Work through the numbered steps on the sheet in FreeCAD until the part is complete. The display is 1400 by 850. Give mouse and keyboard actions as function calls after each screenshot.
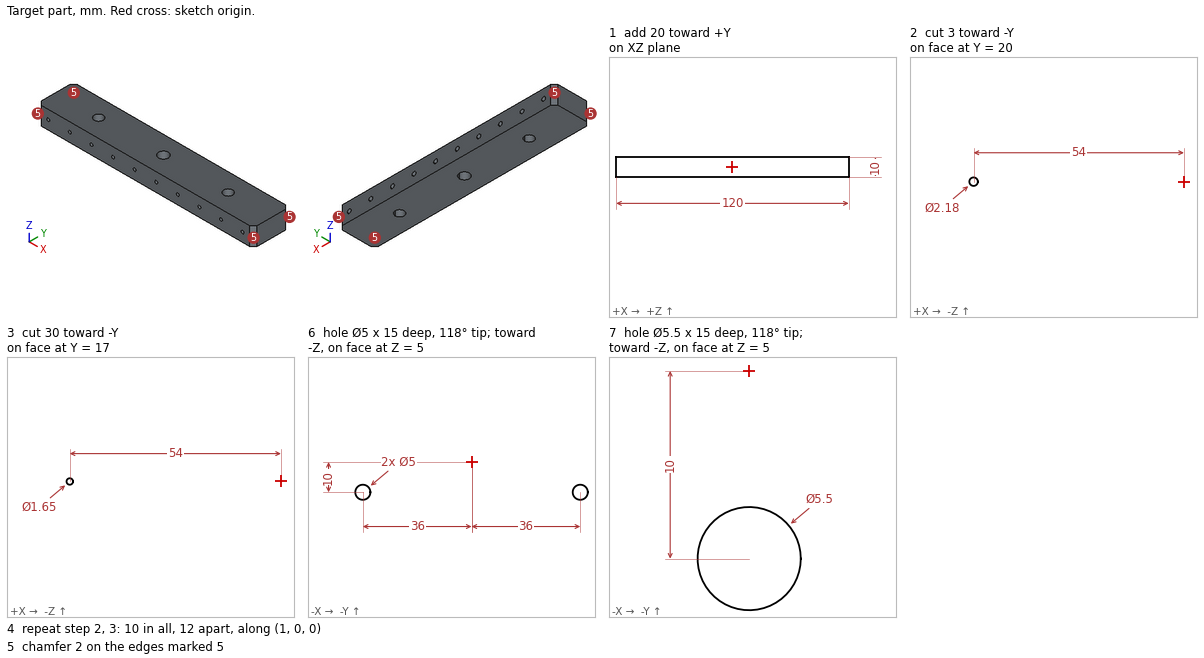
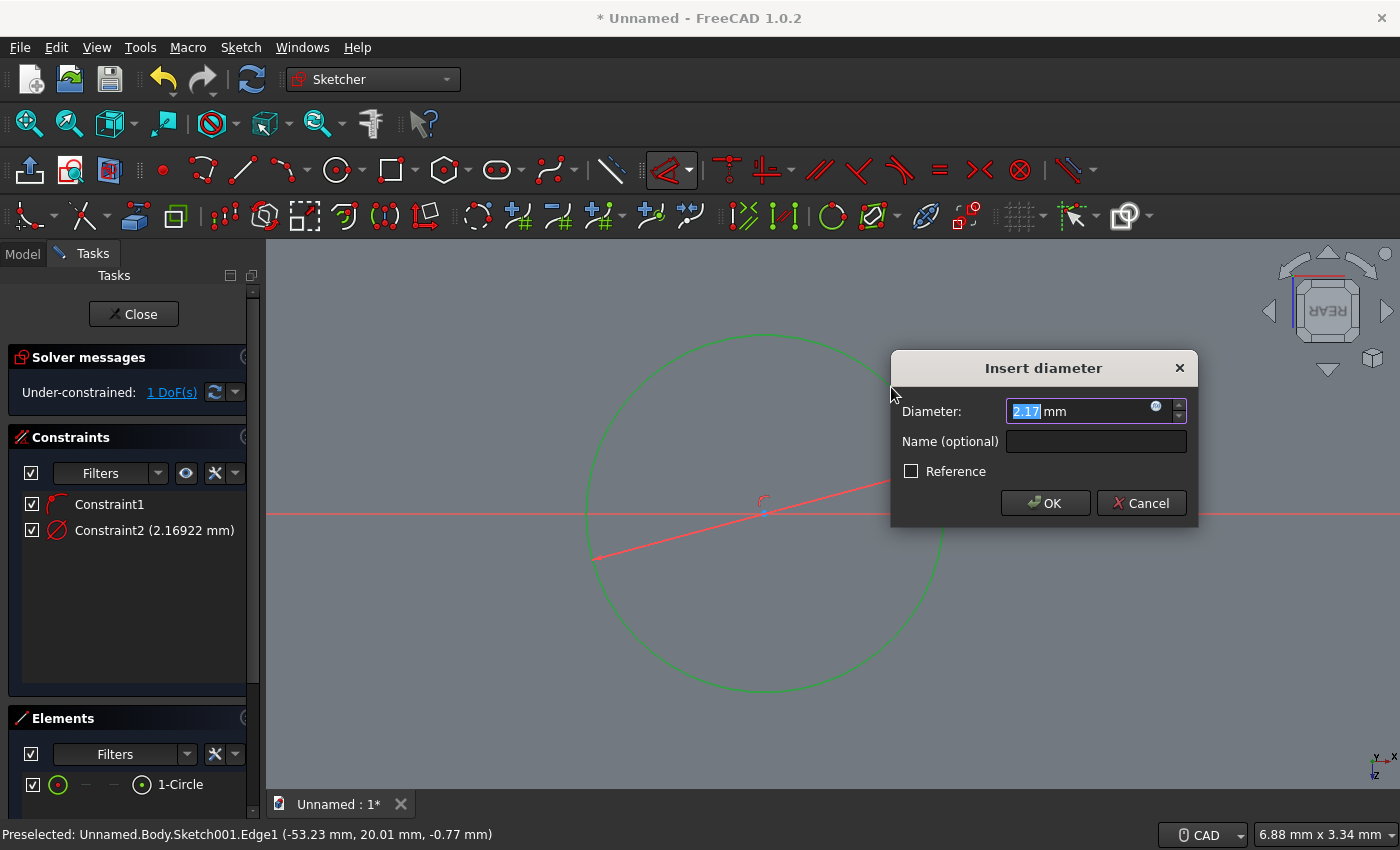
text(2.18)
key(Return)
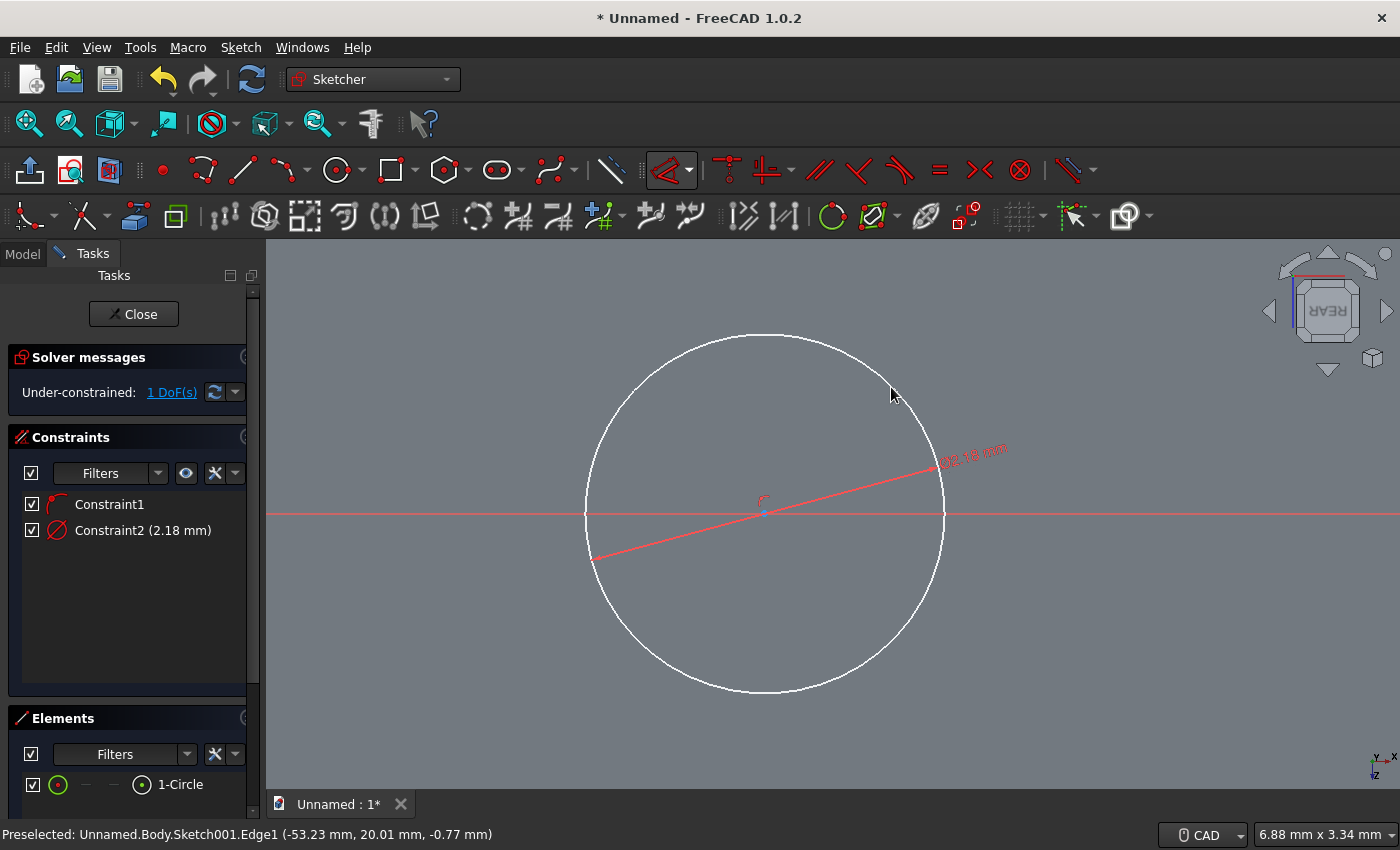
click(765, 514)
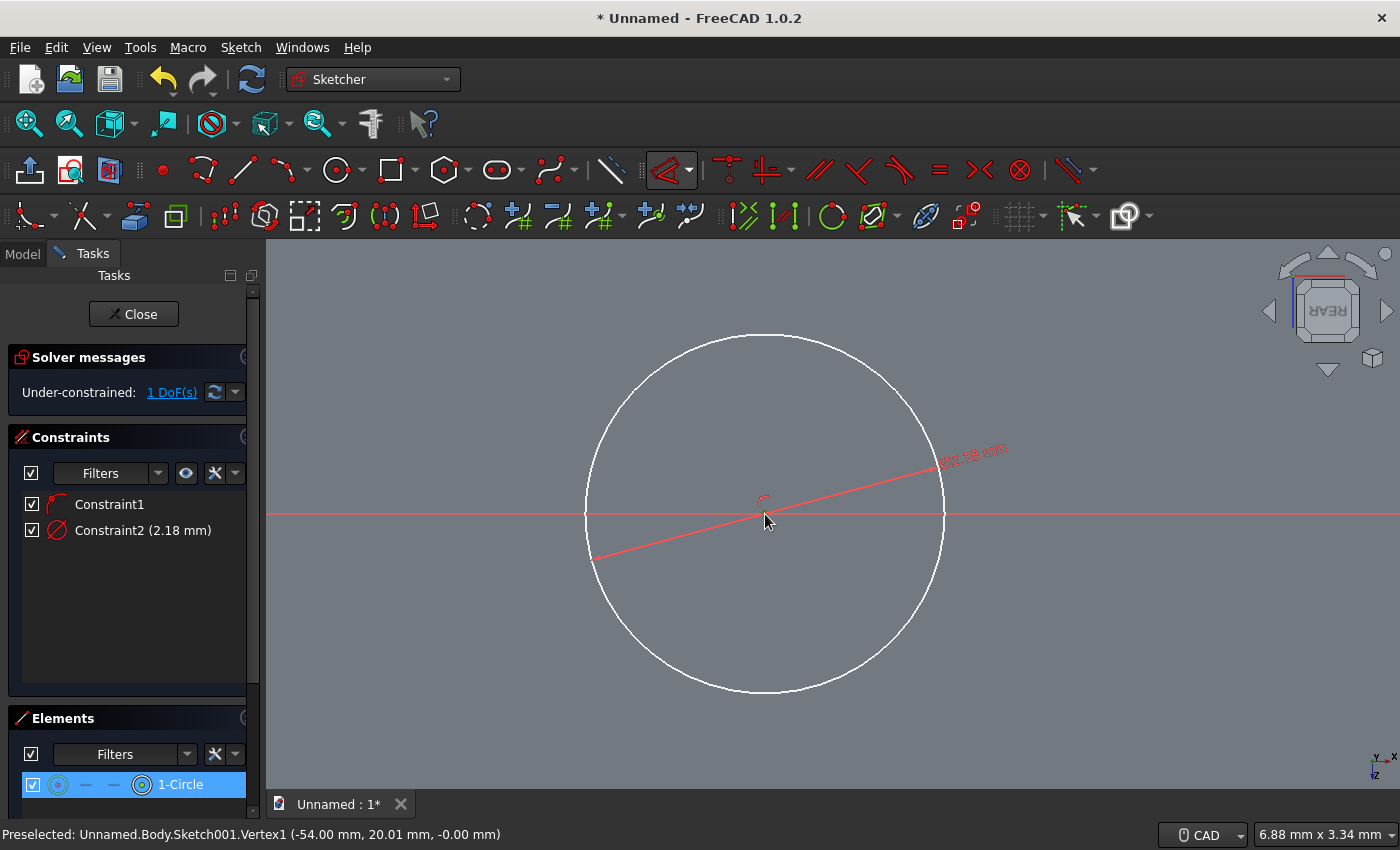
click(692, 170)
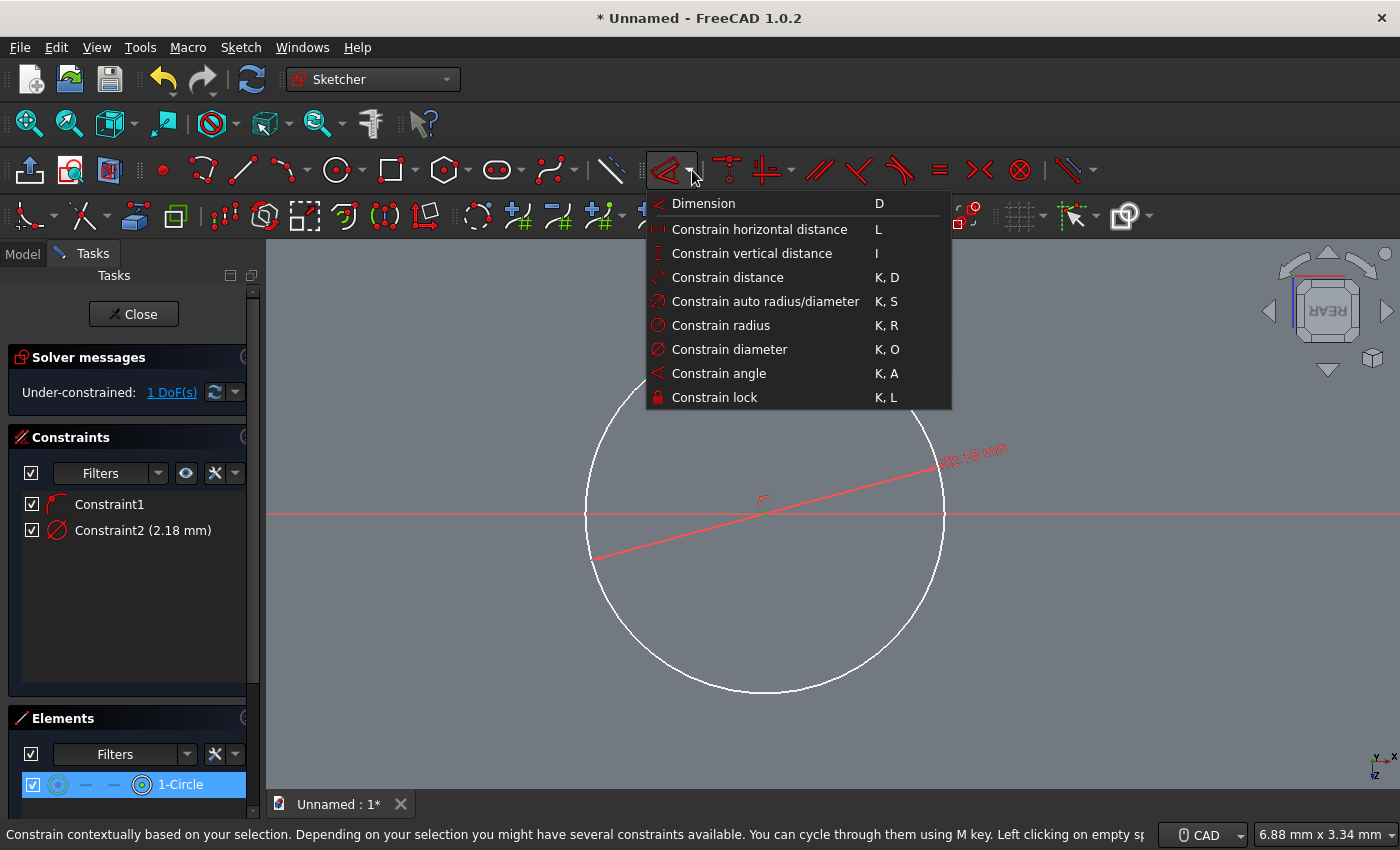
click(799, 229)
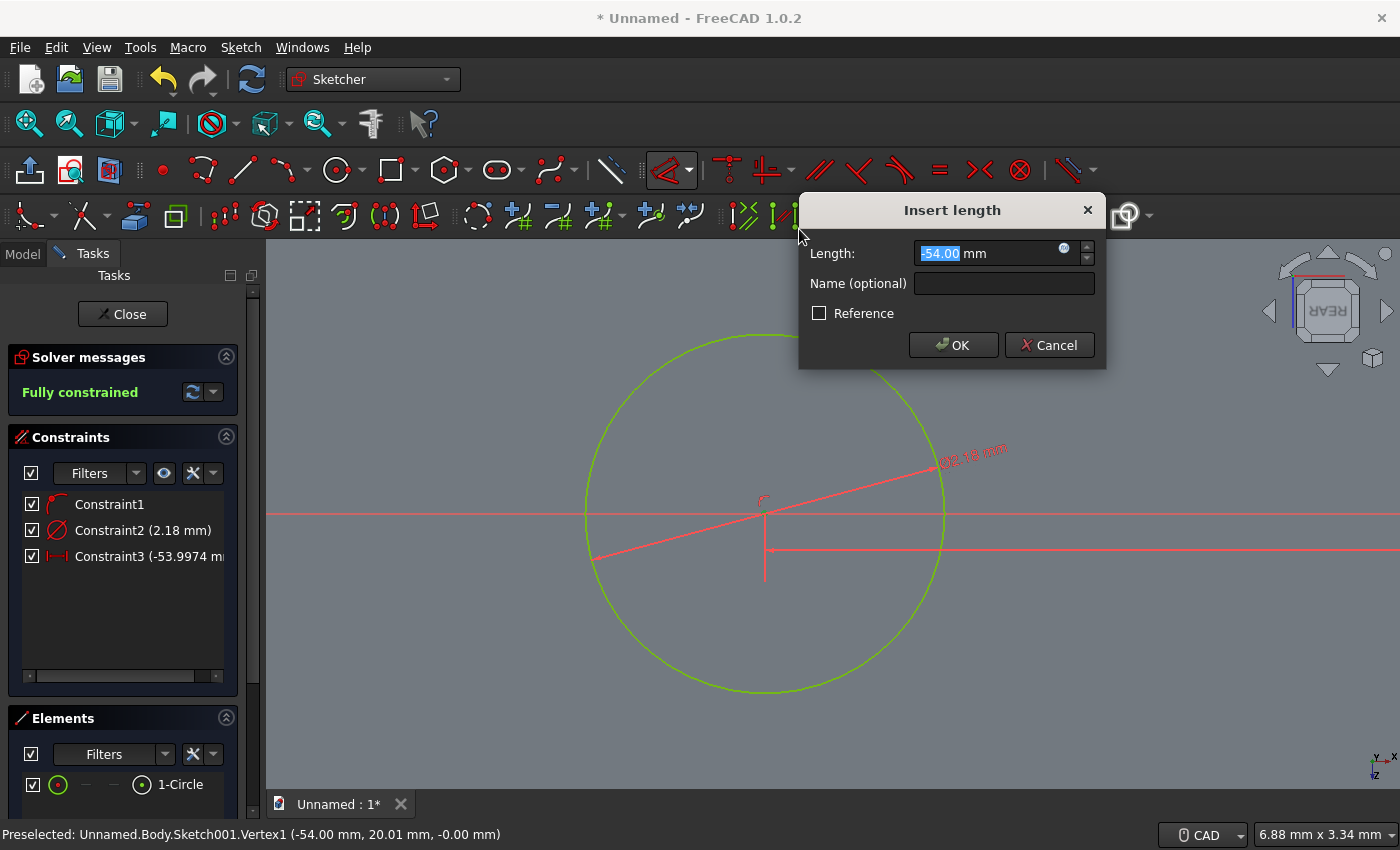
text(-54)
key(Return)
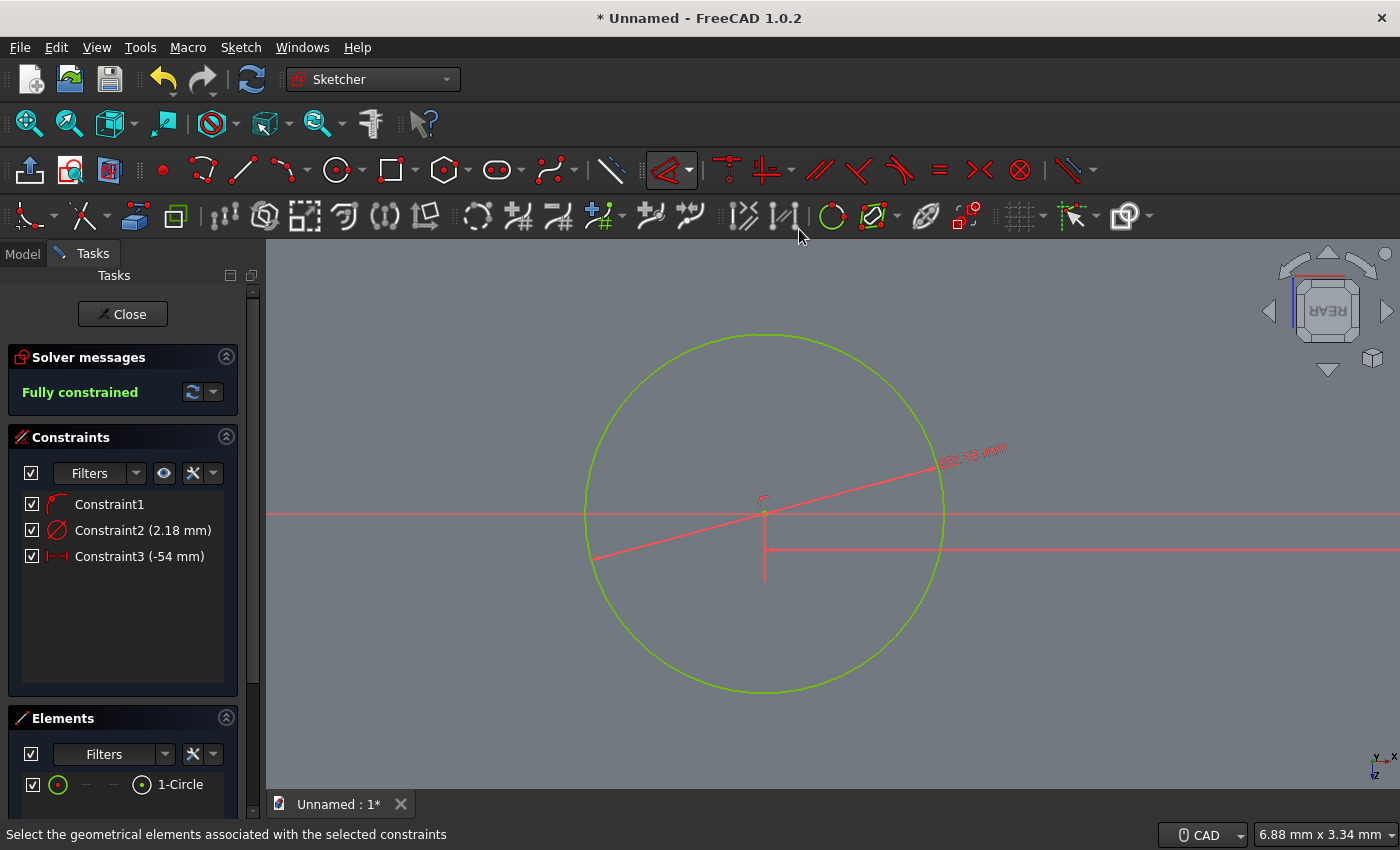
click(123, 314)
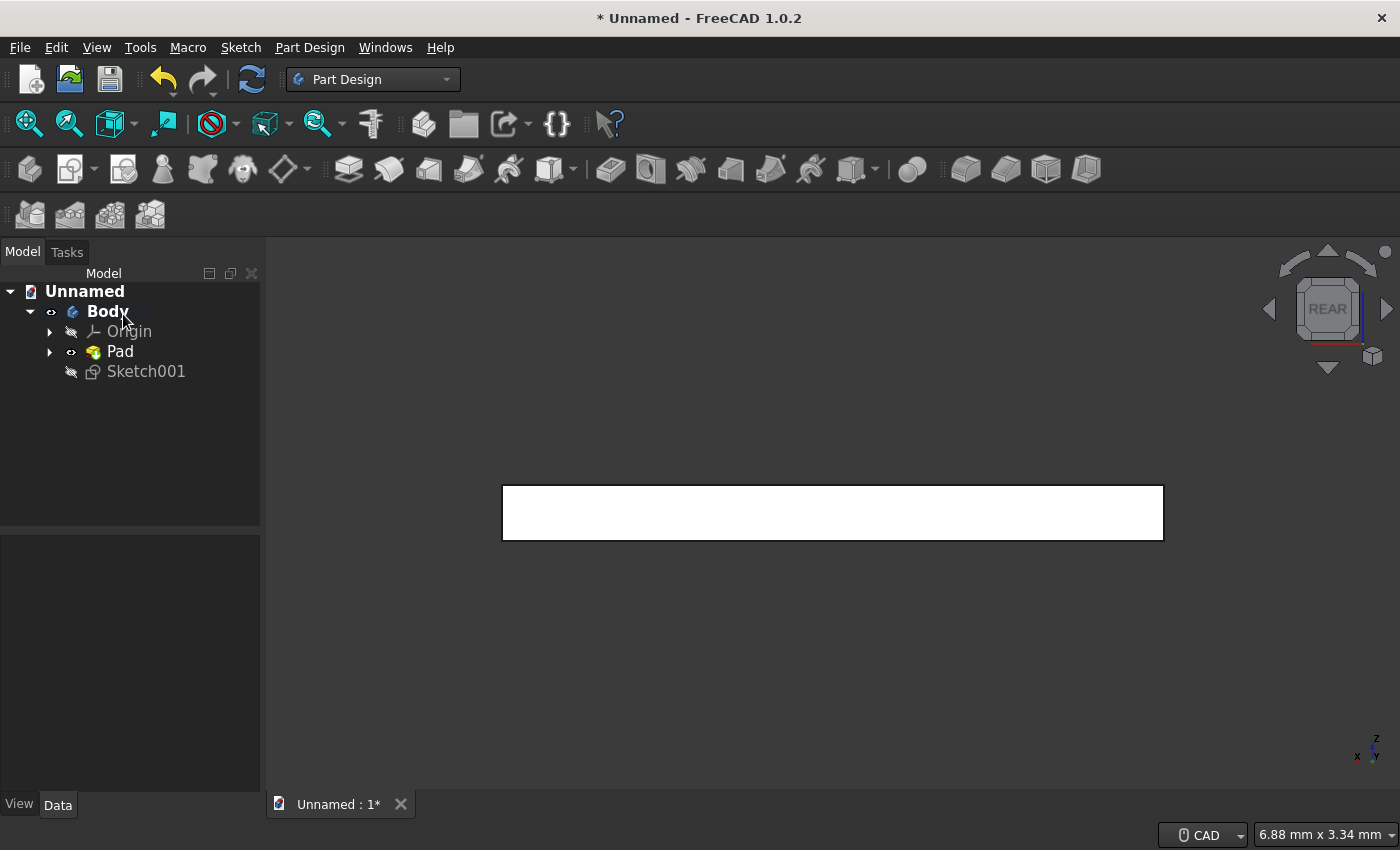
click(612, 170)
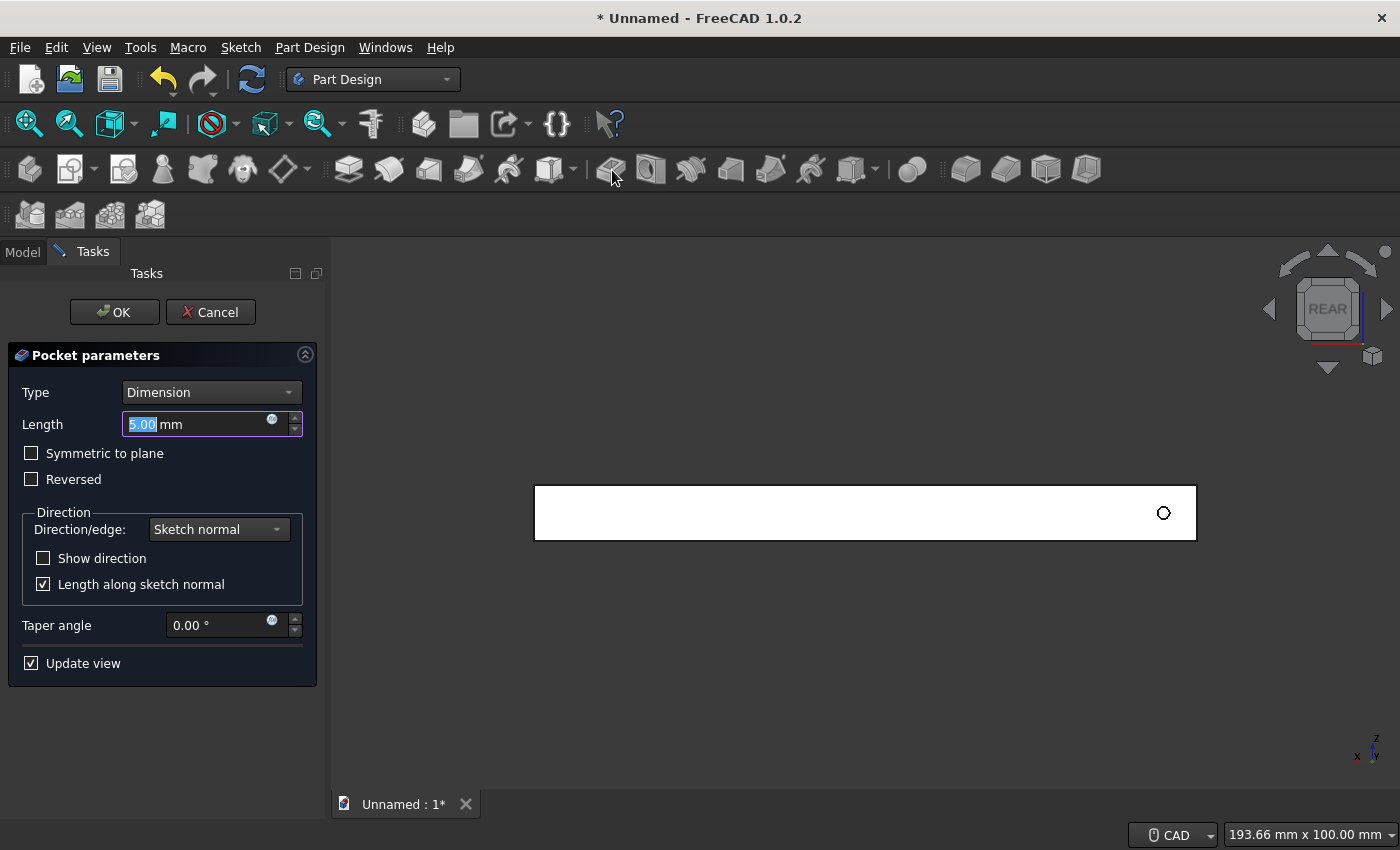
text(3)
key(Tab)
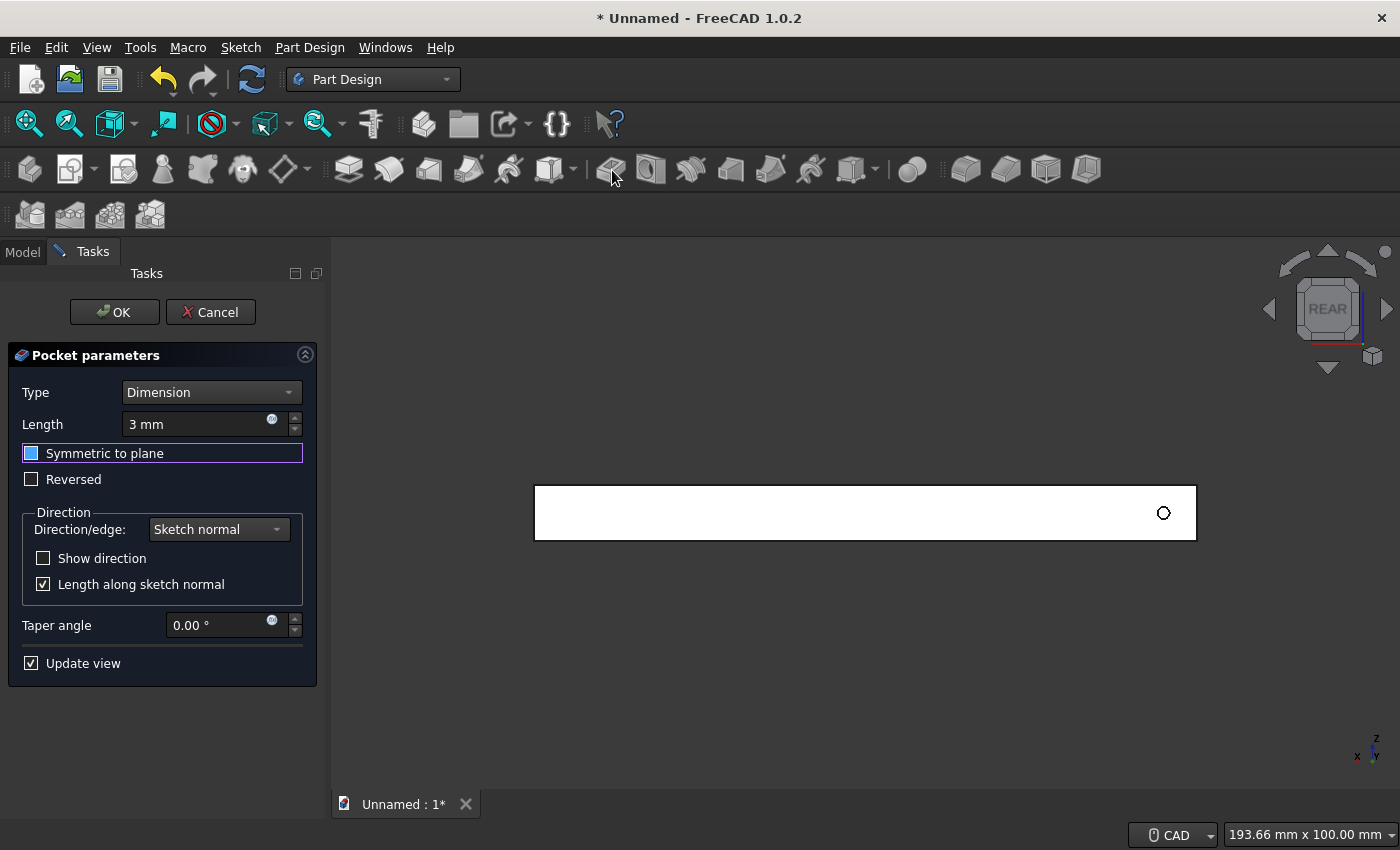
click(115, 312)